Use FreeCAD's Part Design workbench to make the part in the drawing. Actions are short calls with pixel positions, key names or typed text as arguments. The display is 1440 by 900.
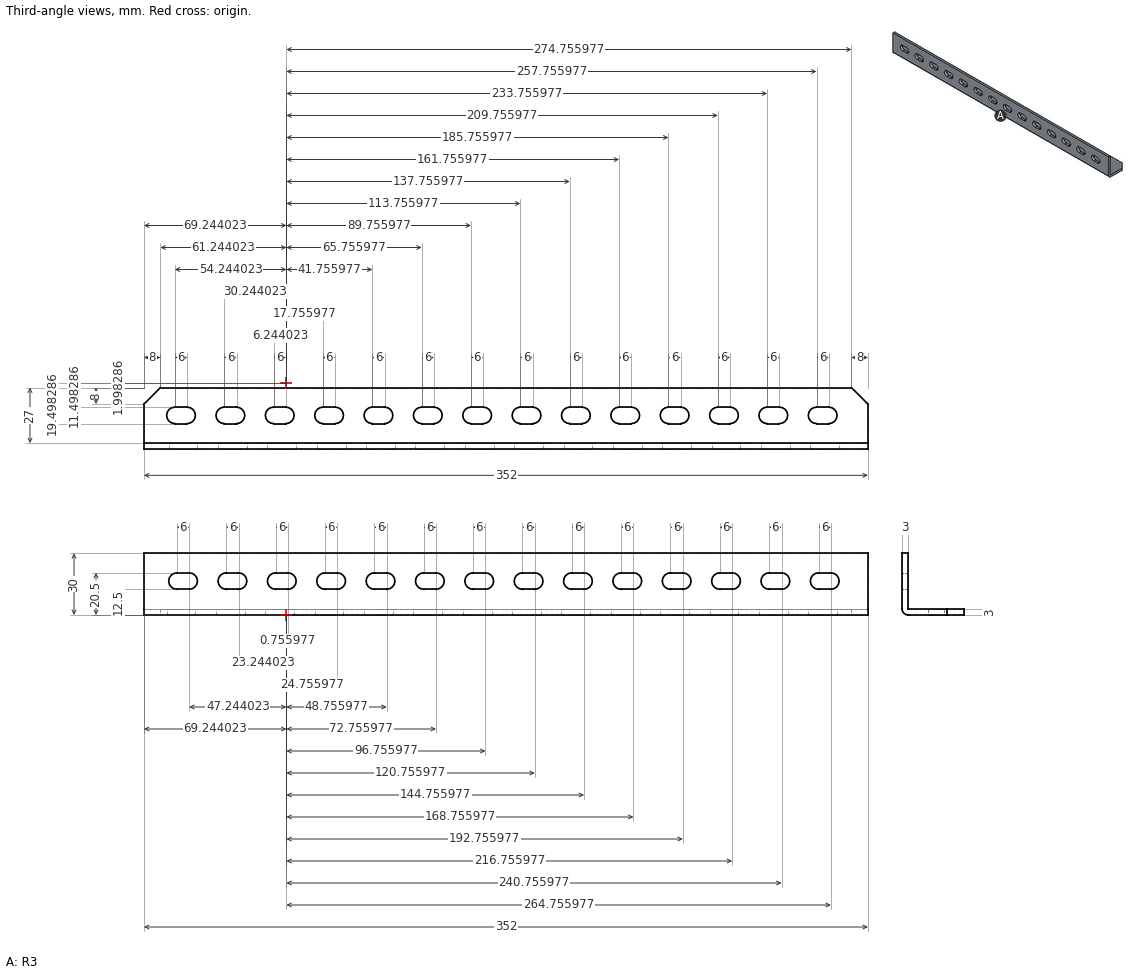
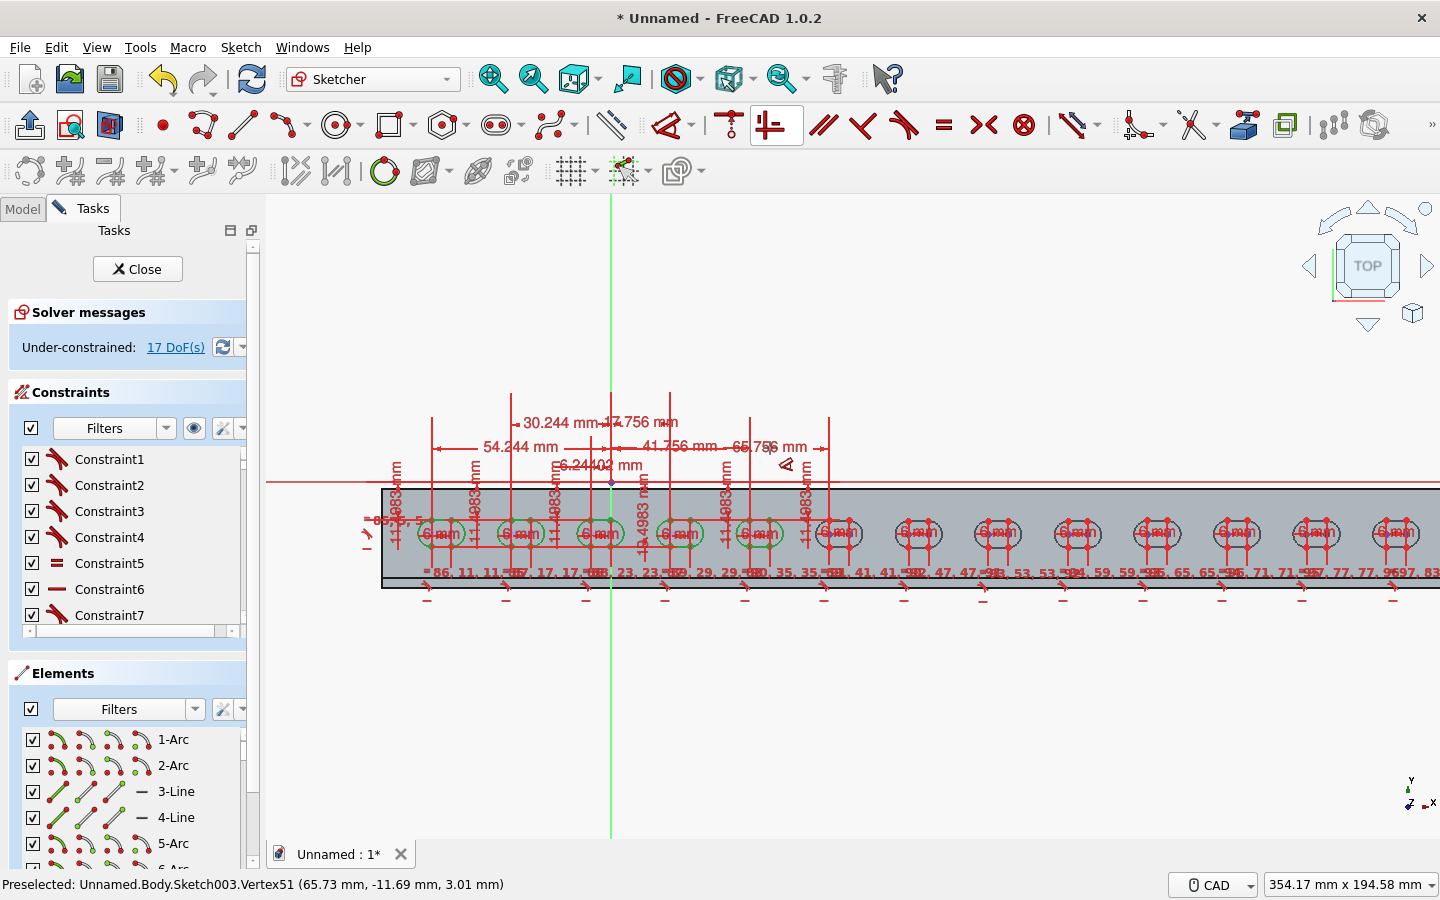
click(829, 521)
click(887, 502)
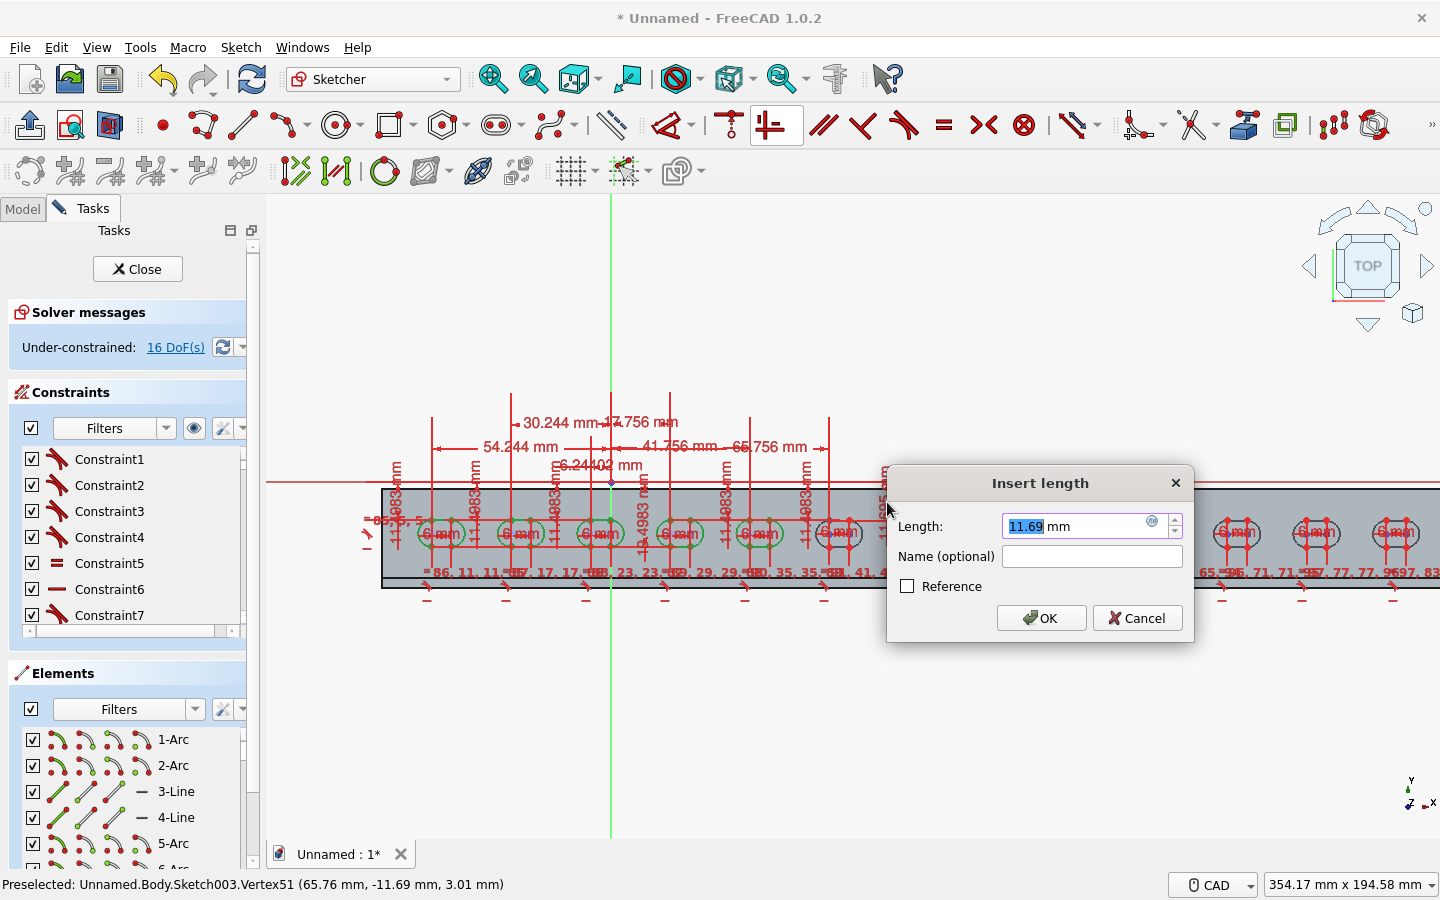
text(11.498286)
key(Return)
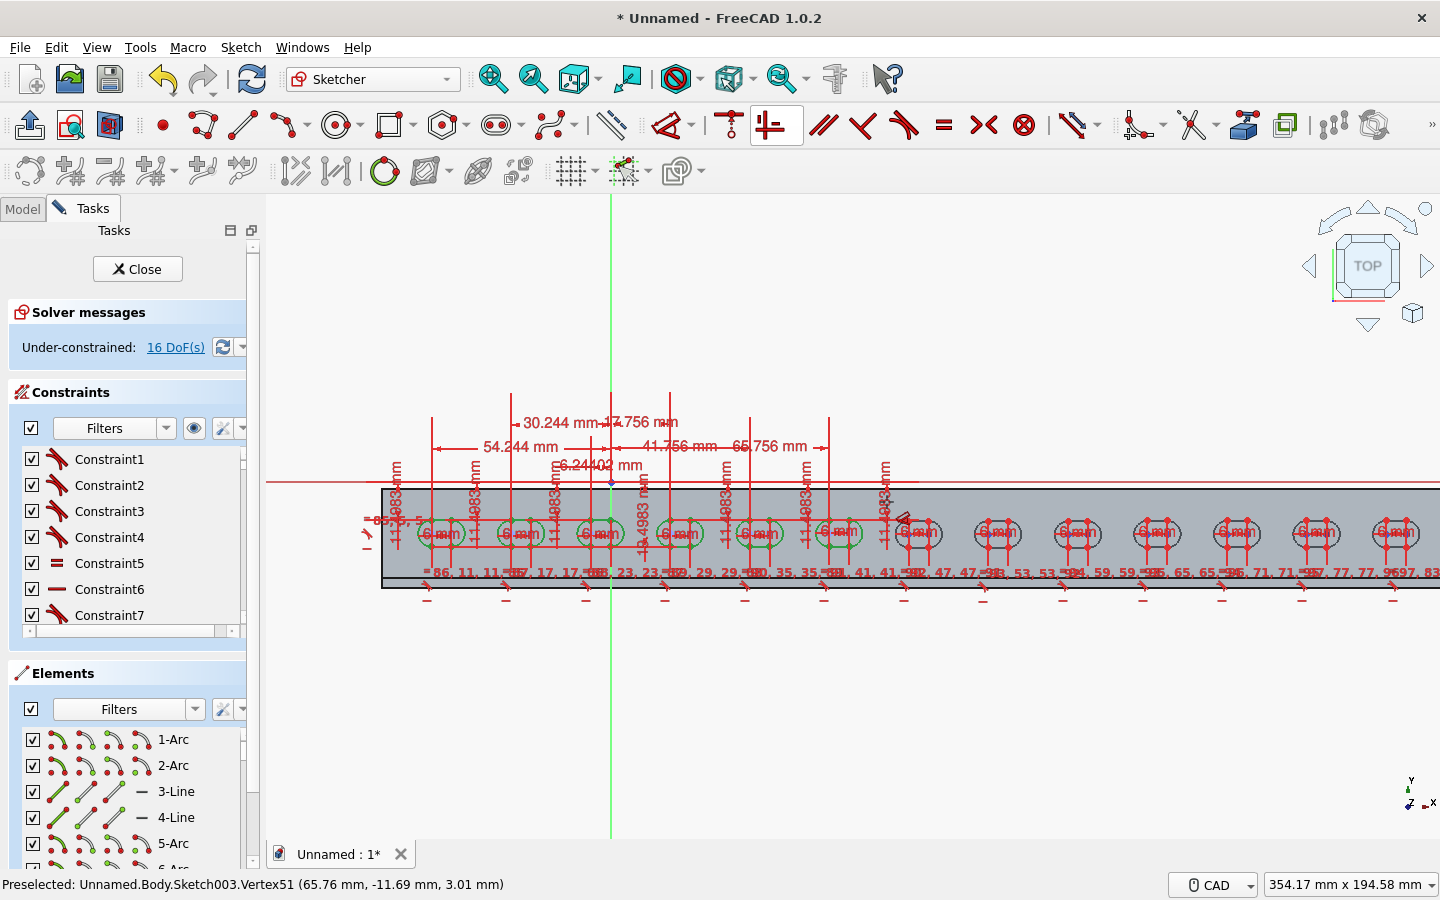
click(909, 521)
click(864, 448)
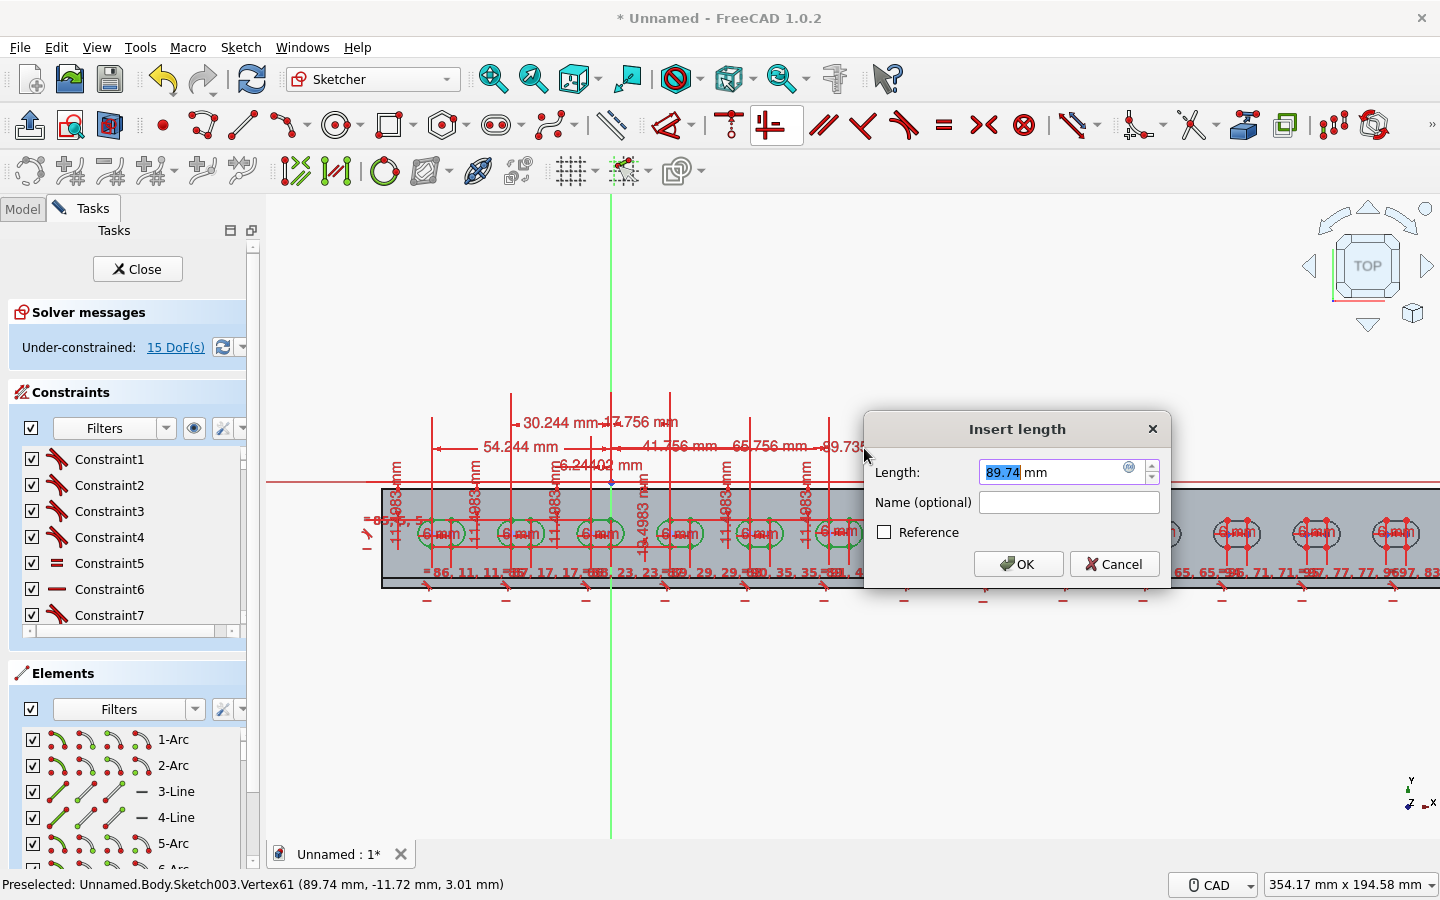
text(89.755977)
key(Return)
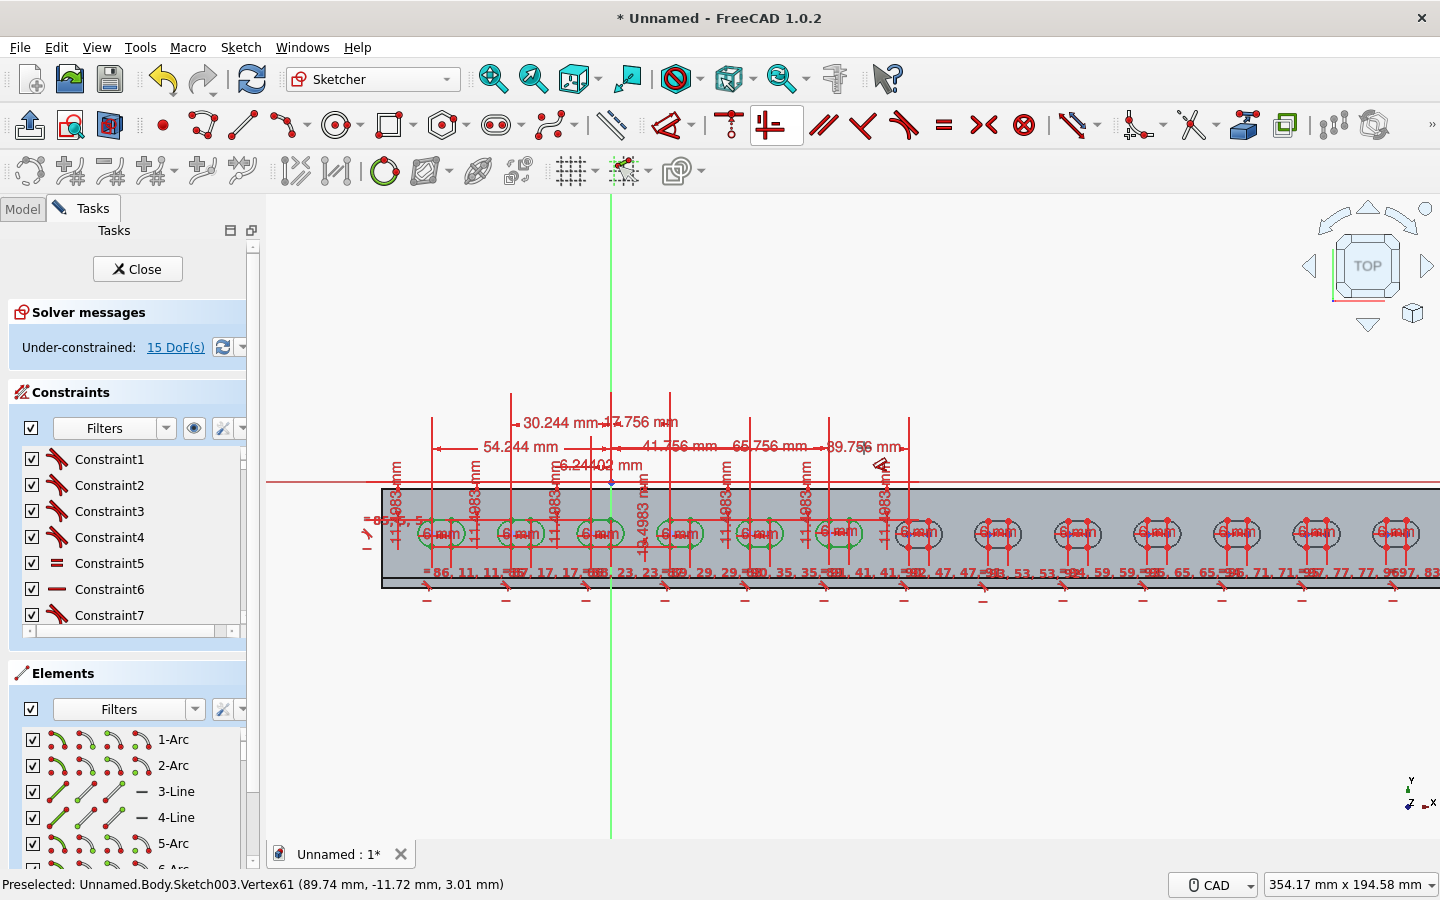
click(909, 521)
click(967, 502)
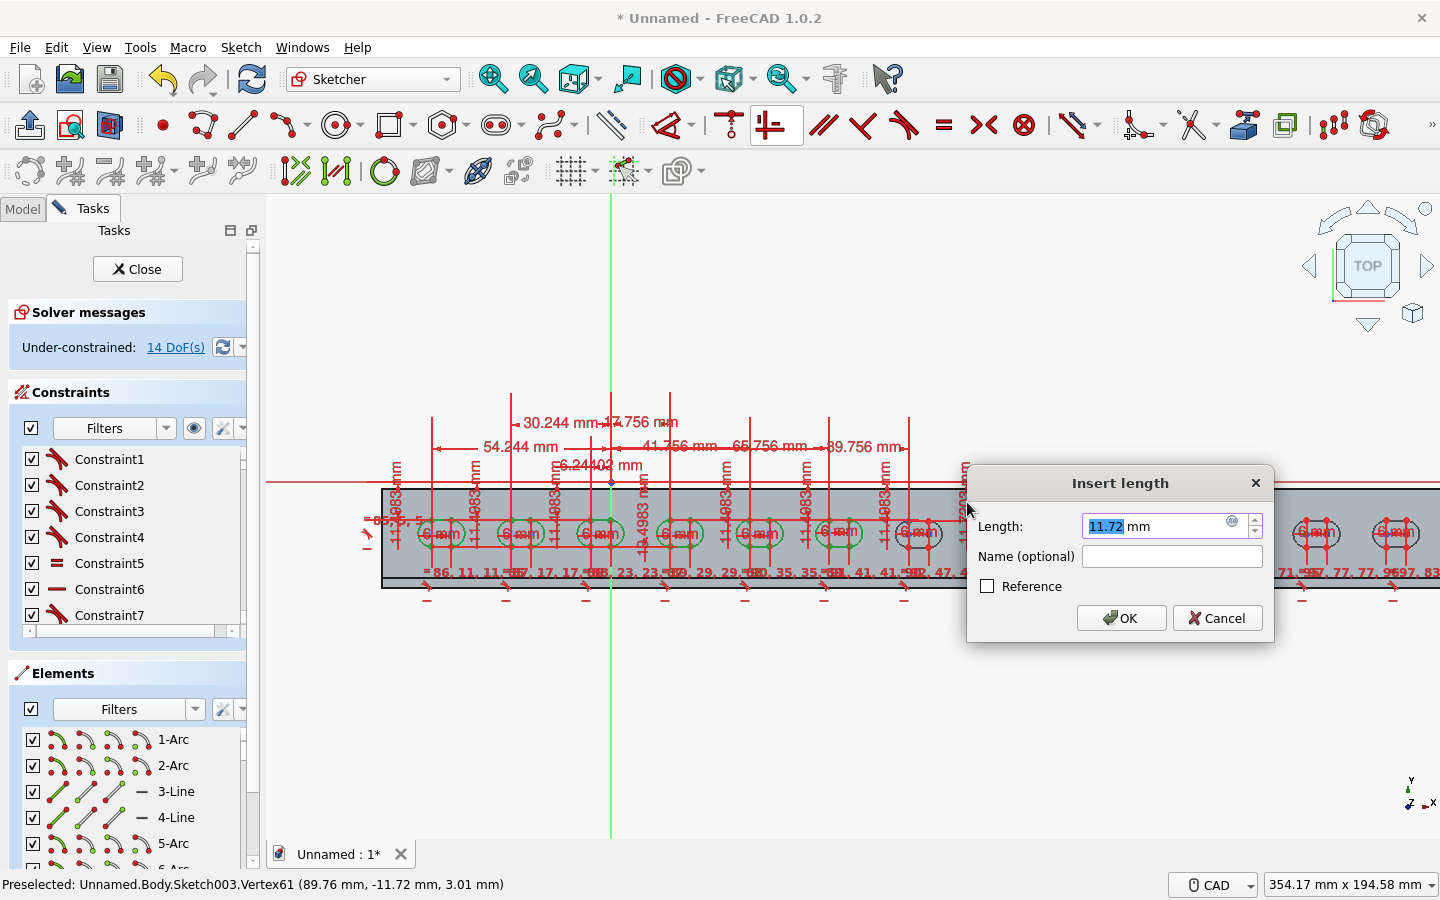
text(11.498286)
key(Return)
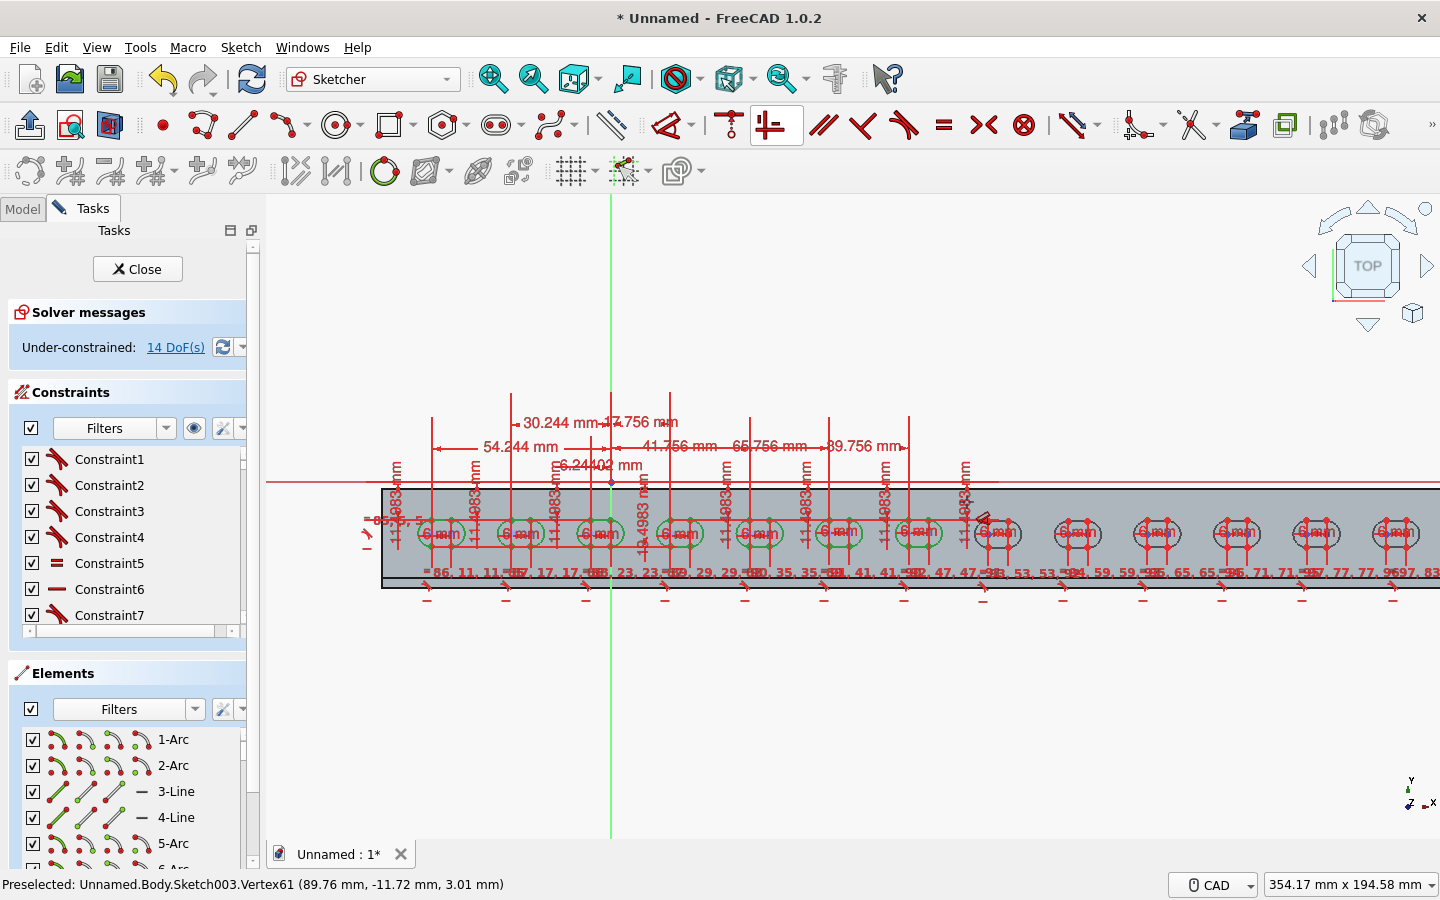
click(988, 521)
click(1046, 502)